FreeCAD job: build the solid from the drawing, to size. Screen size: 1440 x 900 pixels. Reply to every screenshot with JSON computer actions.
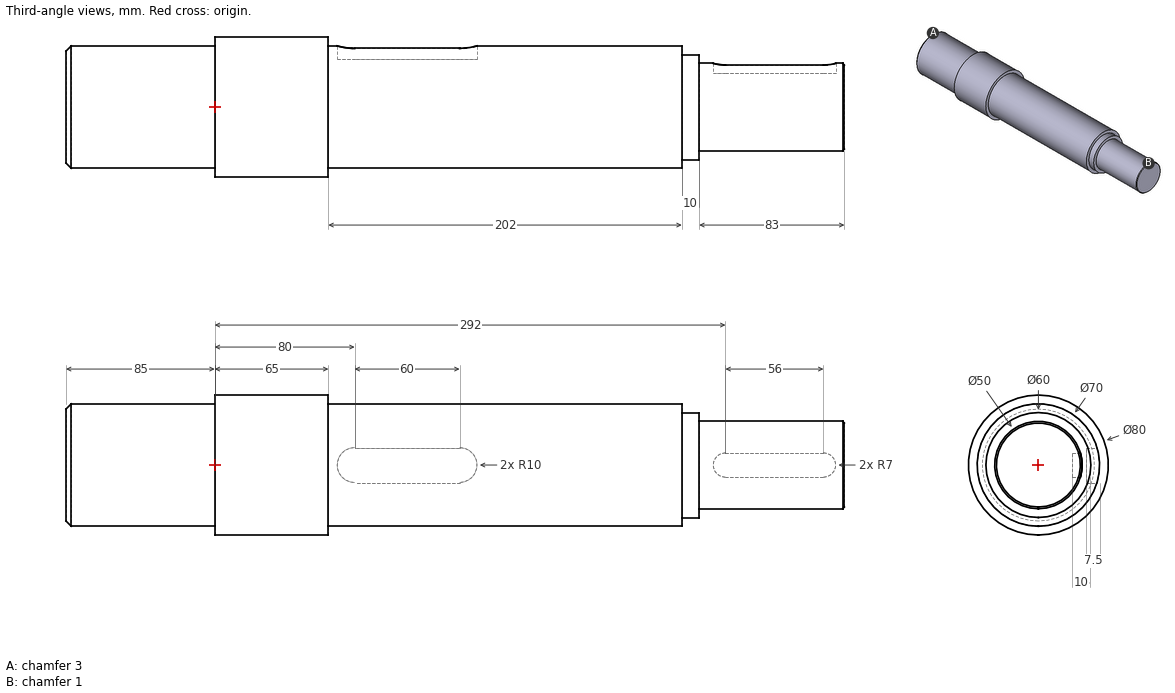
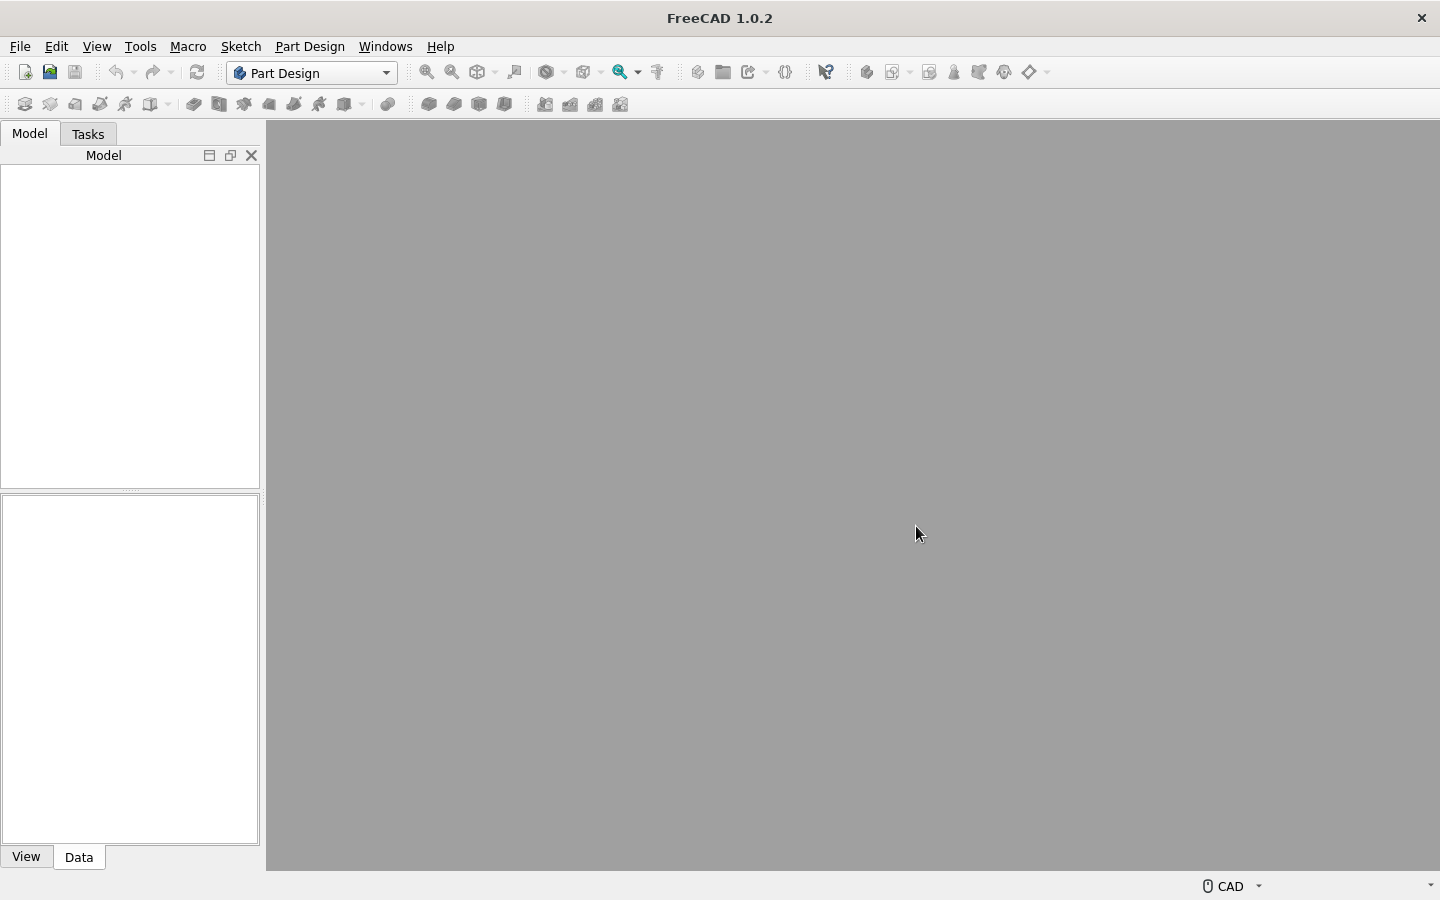
{"action": "left_click", "coordinate": [25, 72]}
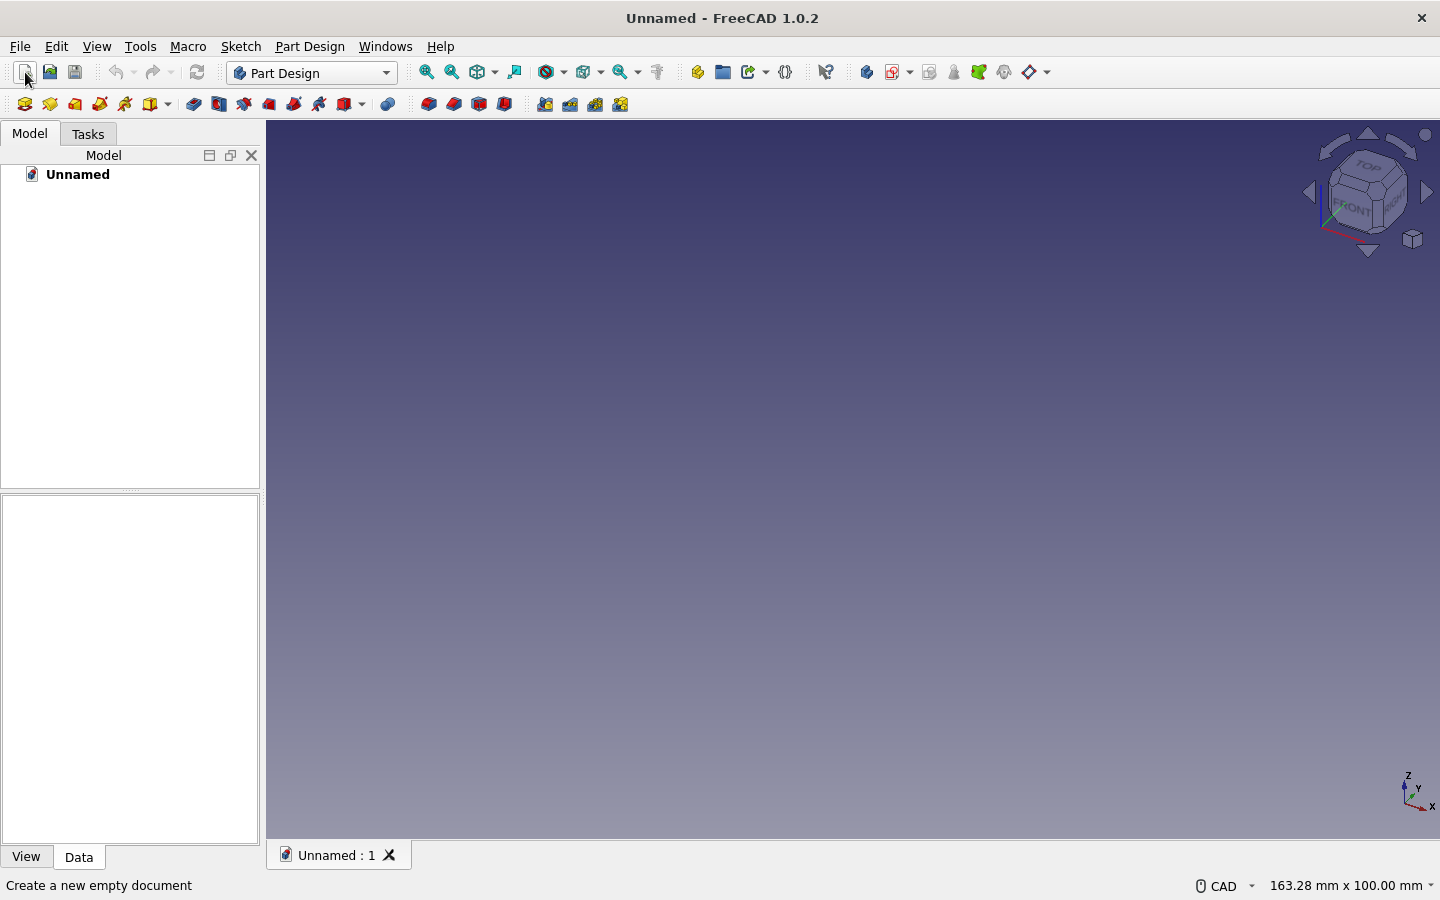
{"action": "left_click", "coordinate": [892, 72]}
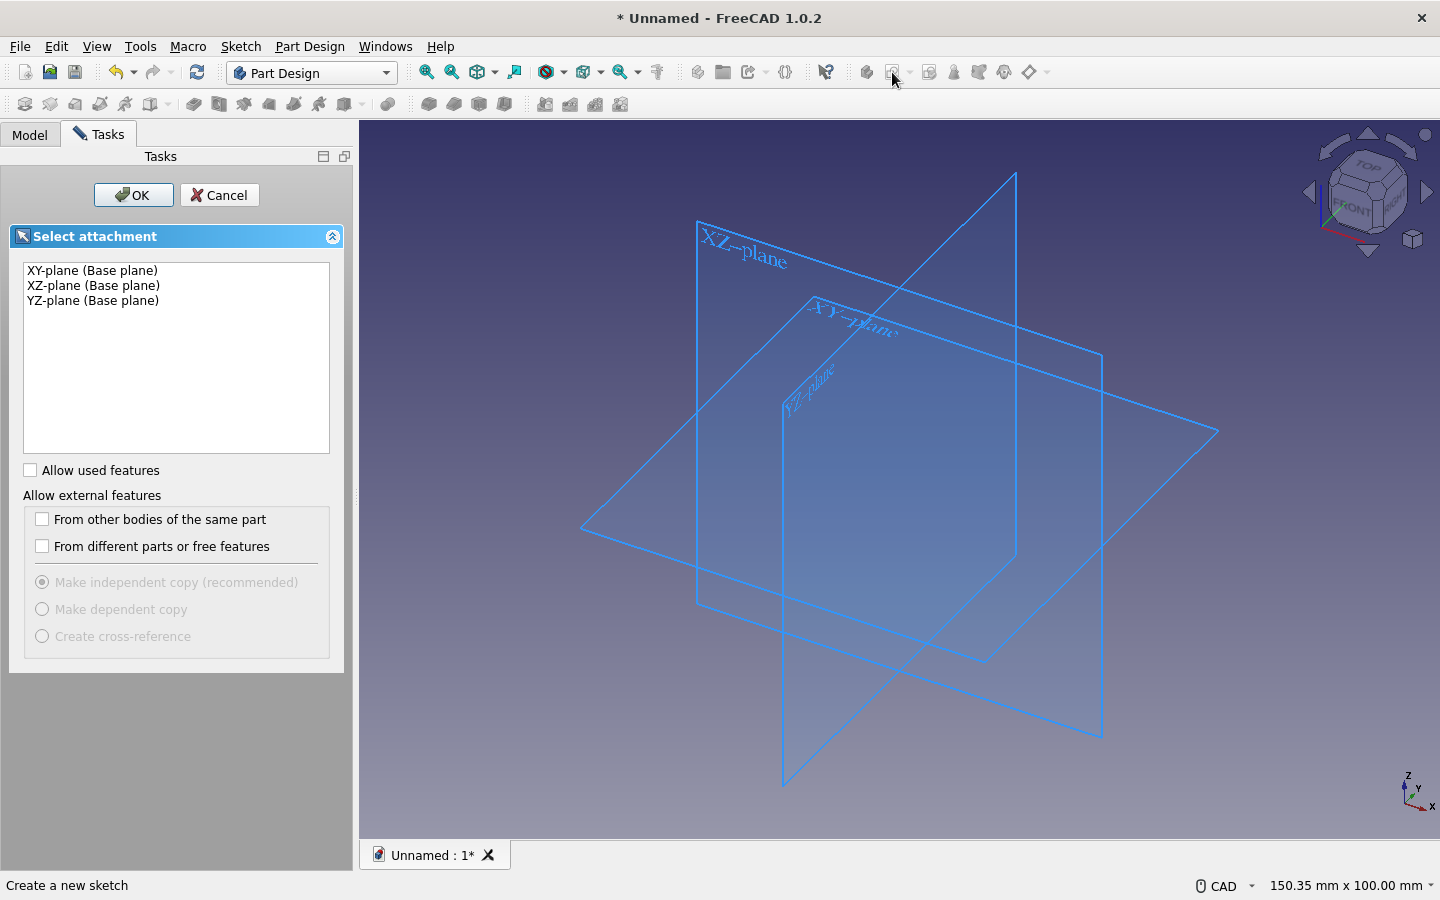
{"action": "left_click", "coordinate": [84, 300]}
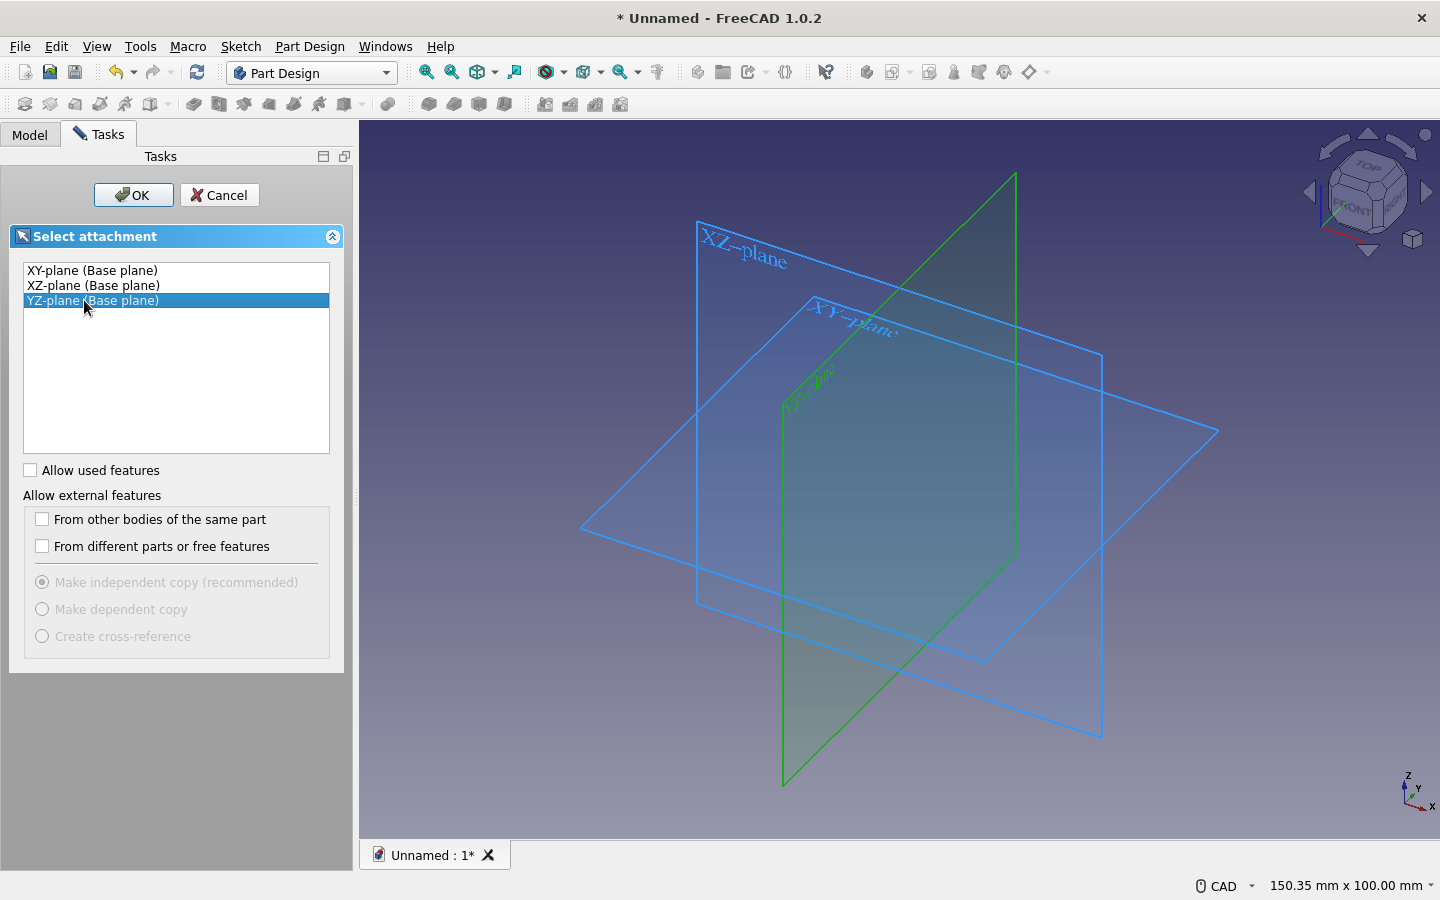
{"action": "left_click", "coordinate": [134, 195]}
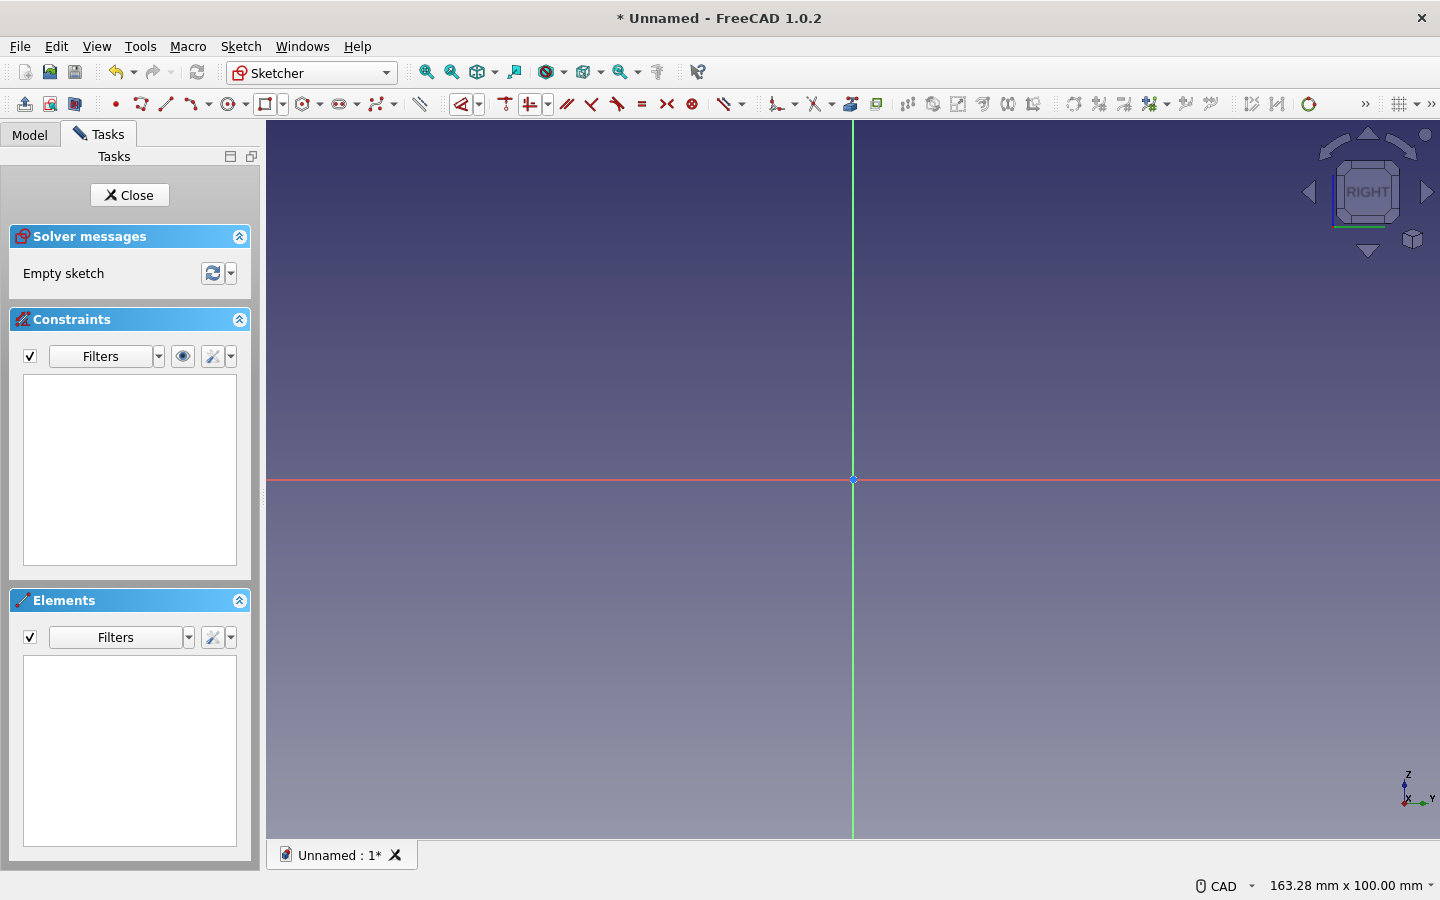
{"action": "key", "text": "g c"}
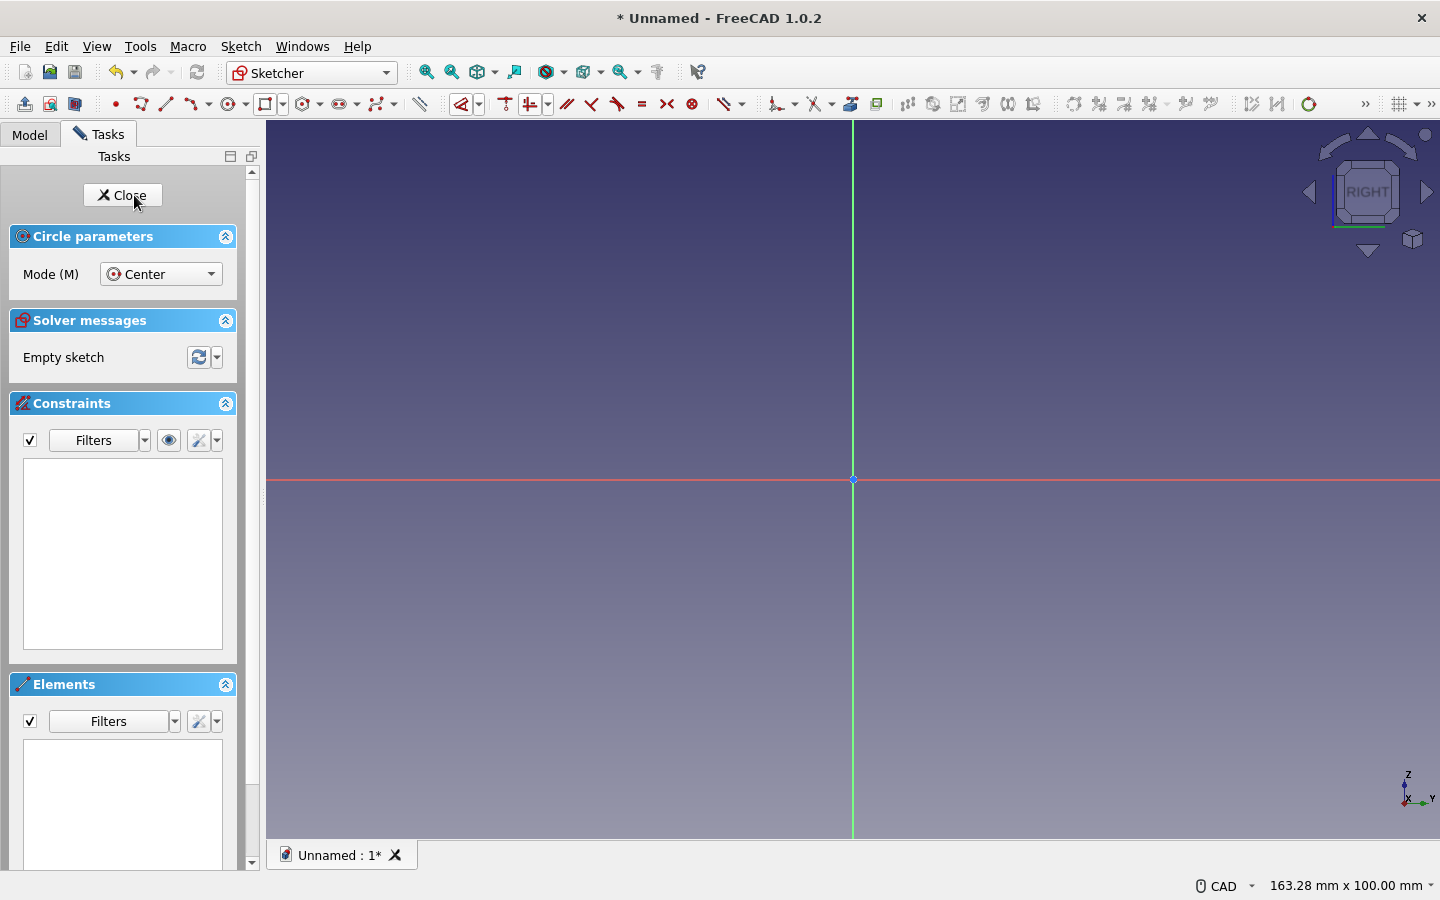
{"action": "left_click", "coordinate": [853, 480]}
{"action": "left_click", "coordinate": [1056, 276]}
{"action": "key", "text": "Escape"}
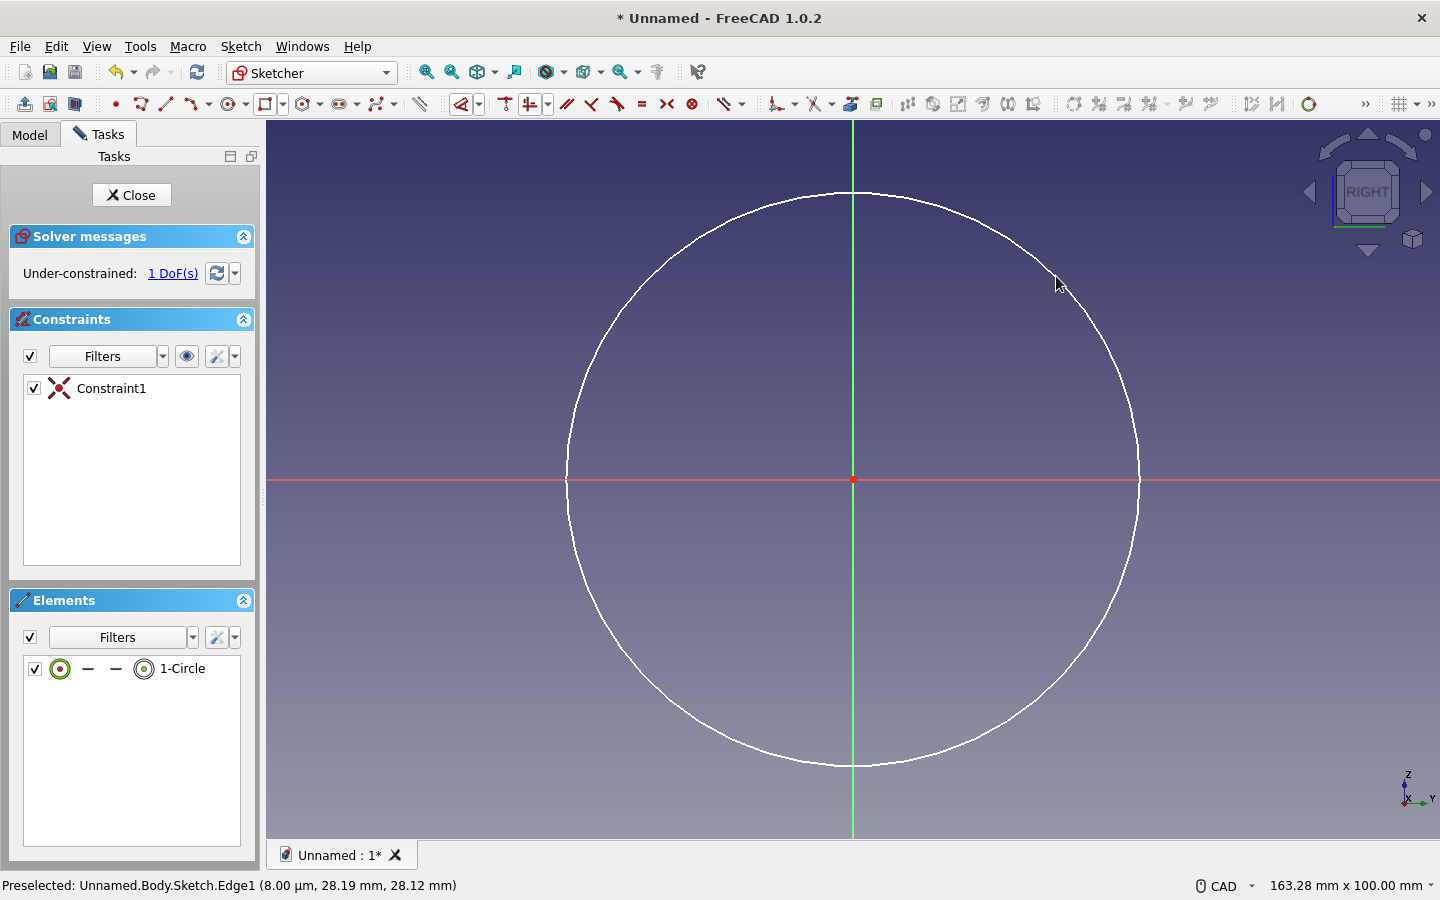
{"action": "key", "text": "d"}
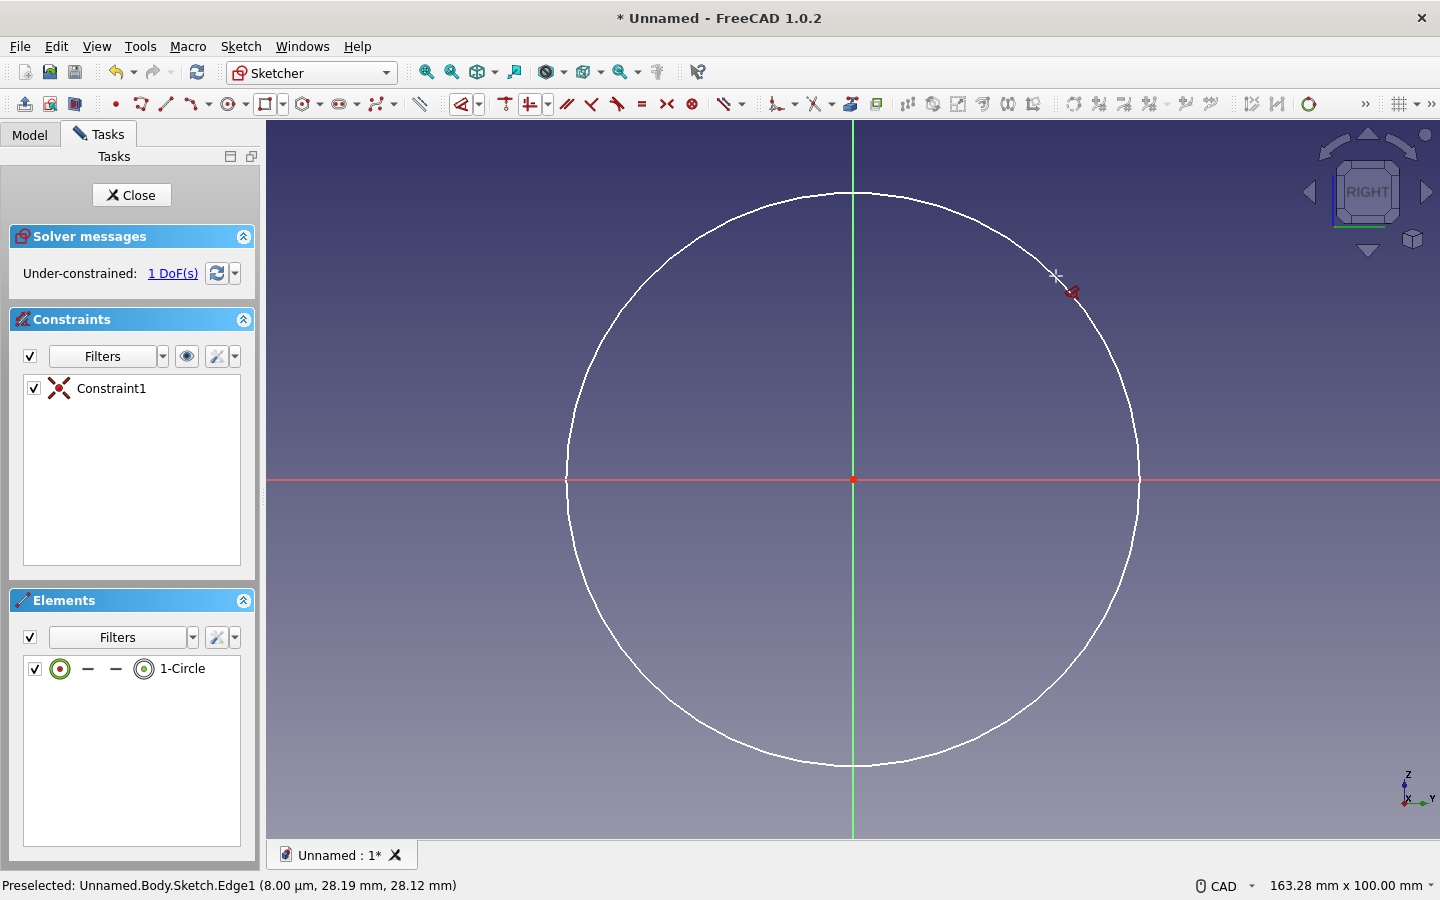
{"action": "left_click", "coordinate": [1055, 276]}
{"action": "left_click", "coordinate": [1078, 253]}